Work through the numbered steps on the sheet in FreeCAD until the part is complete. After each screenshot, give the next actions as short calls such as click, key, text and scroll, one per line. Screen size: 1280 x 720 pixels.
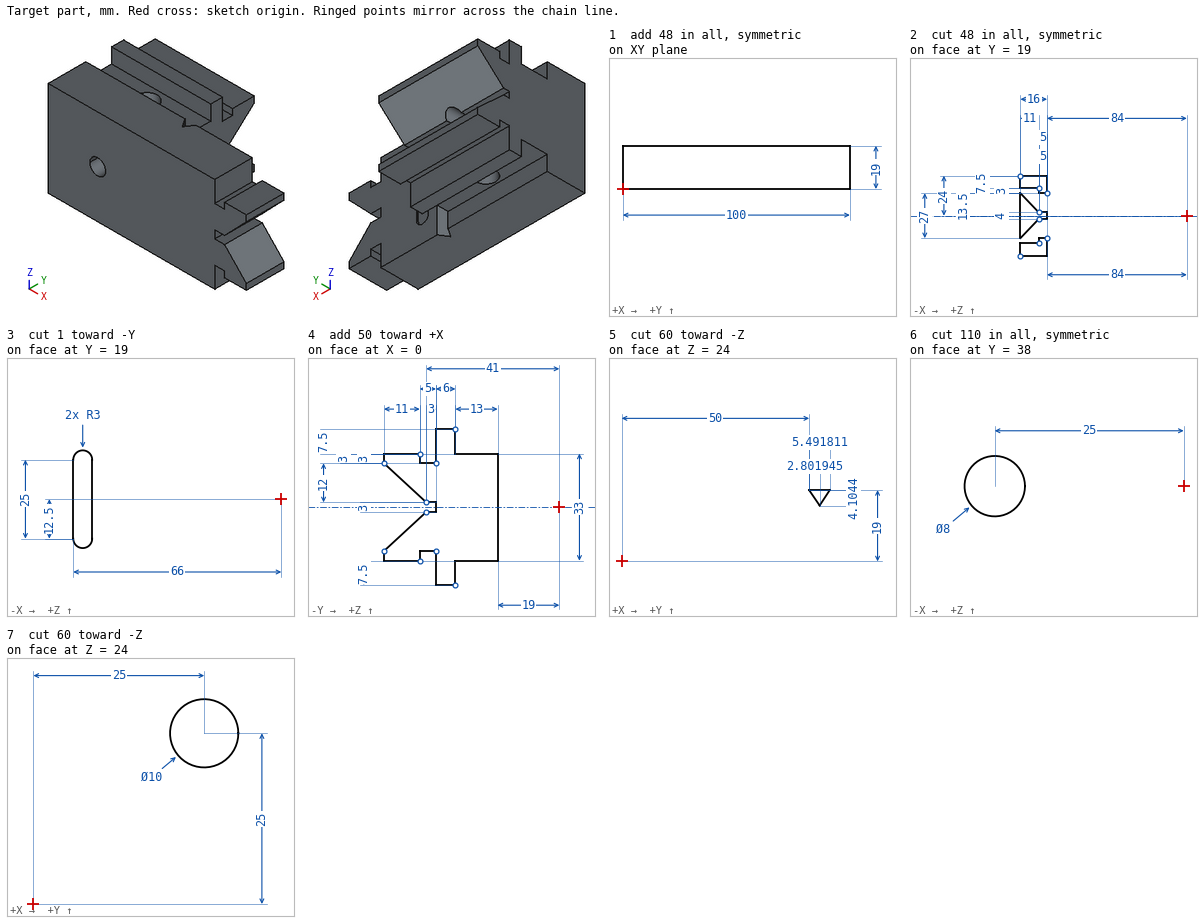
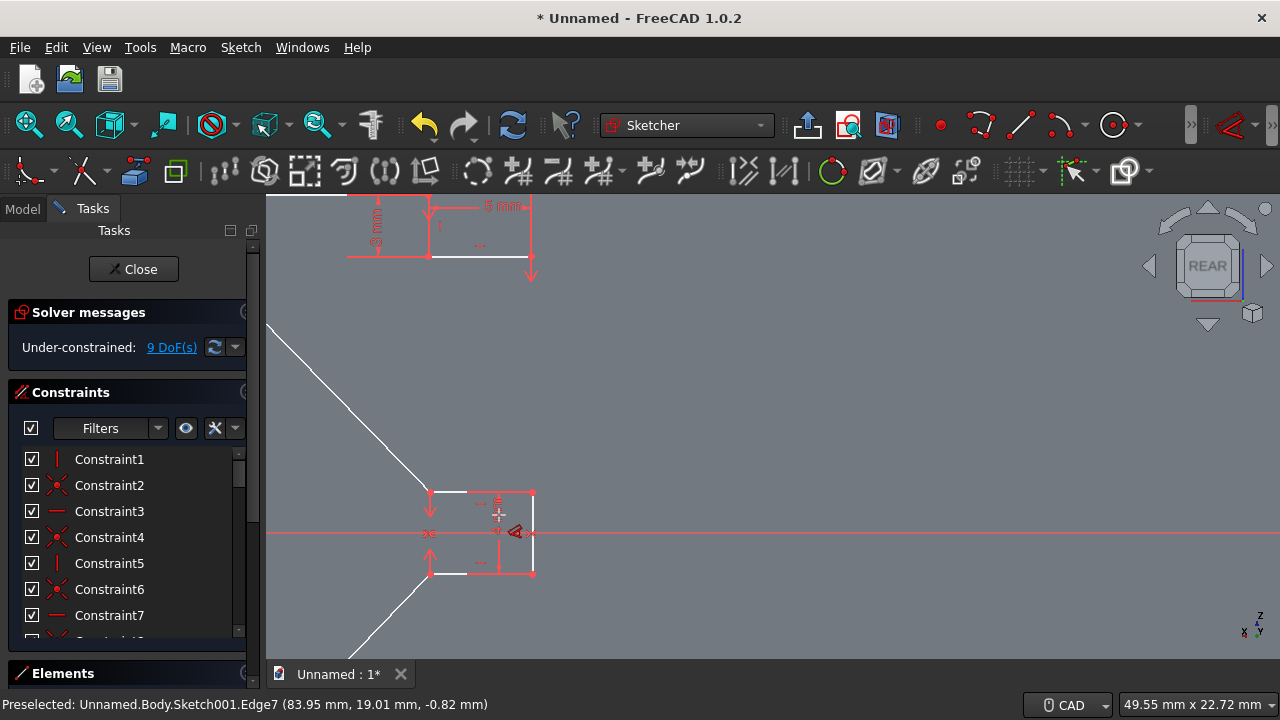
click(502, 492)
click(481, 458)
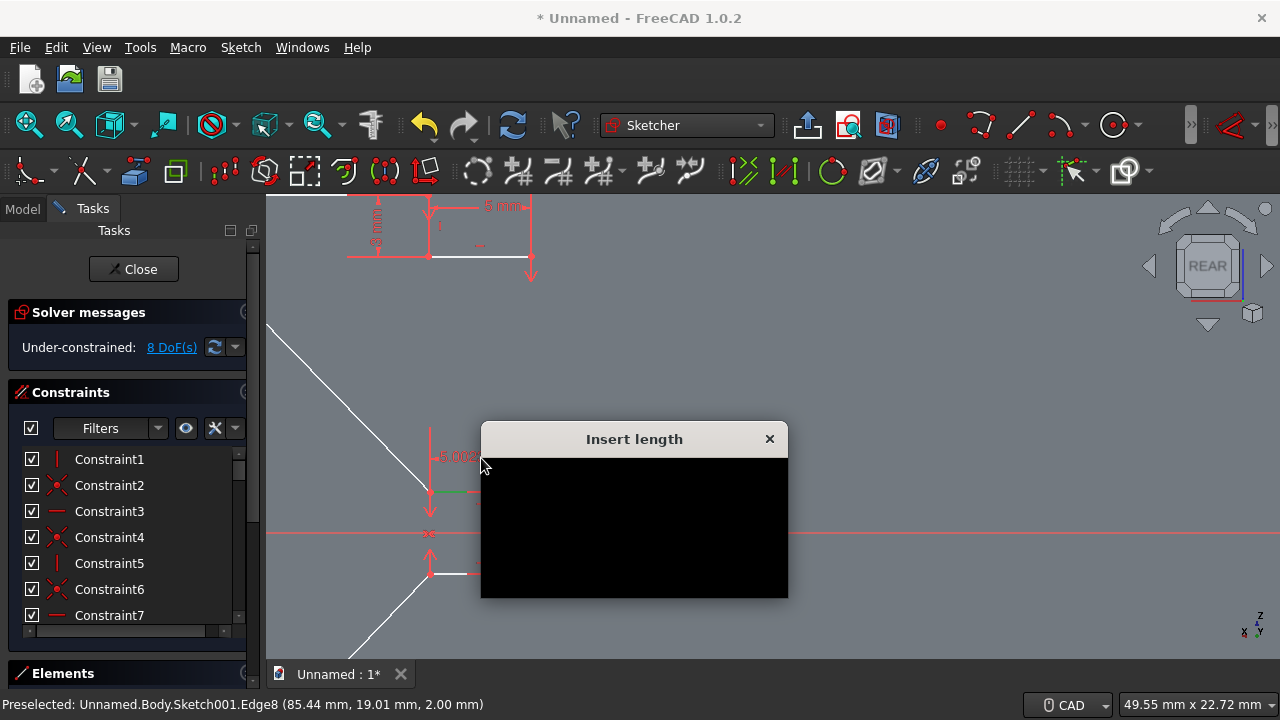
text(5)
key(Return)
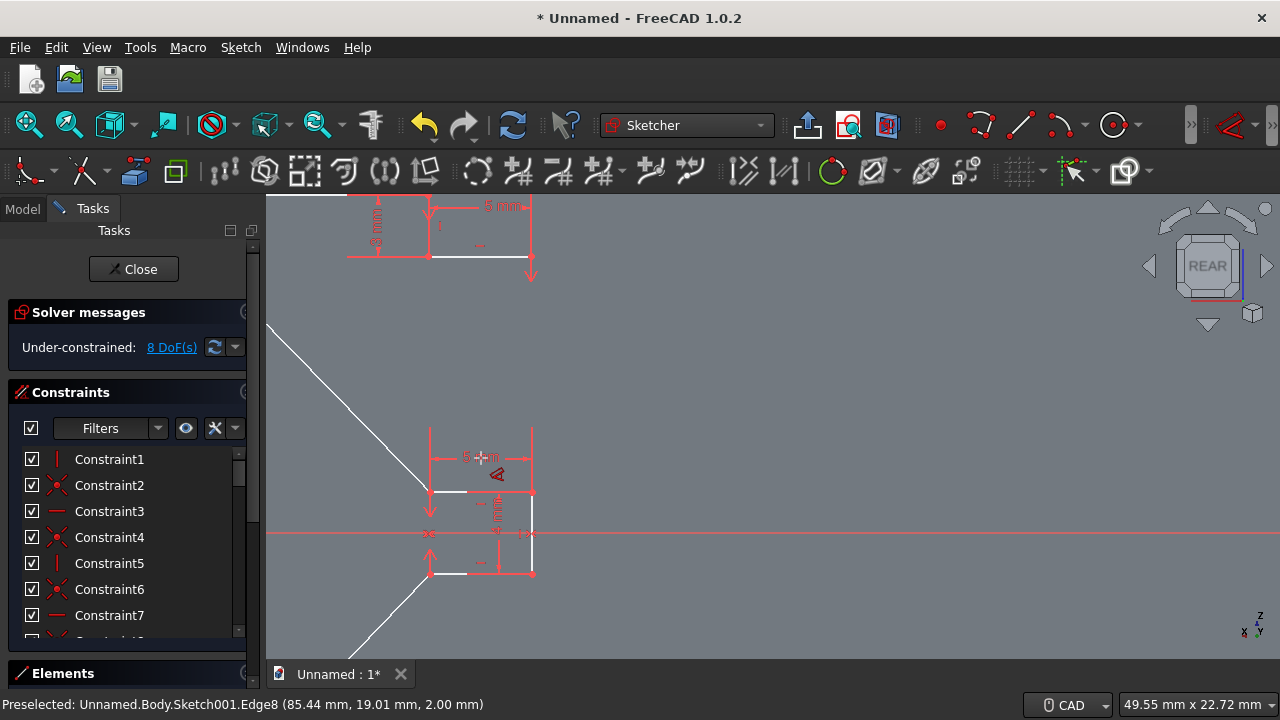
scroll(479, 381, down, 6)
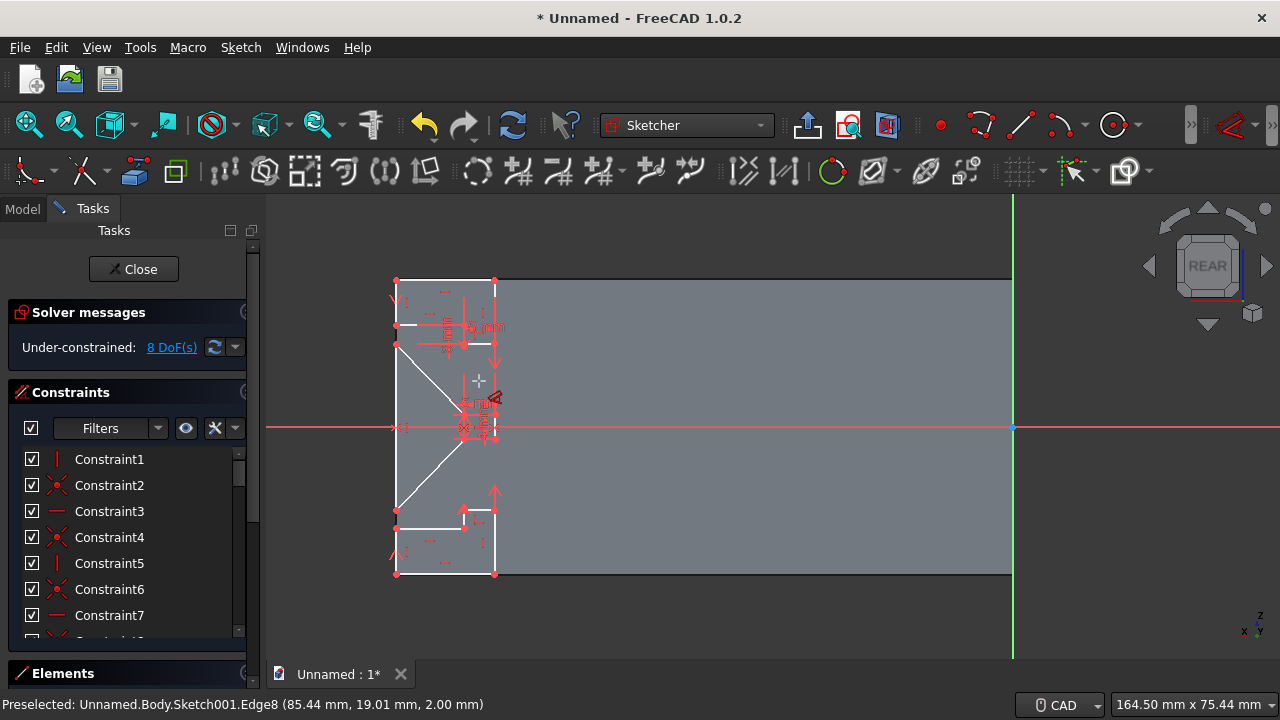
click(465, 280)
click(445, 246)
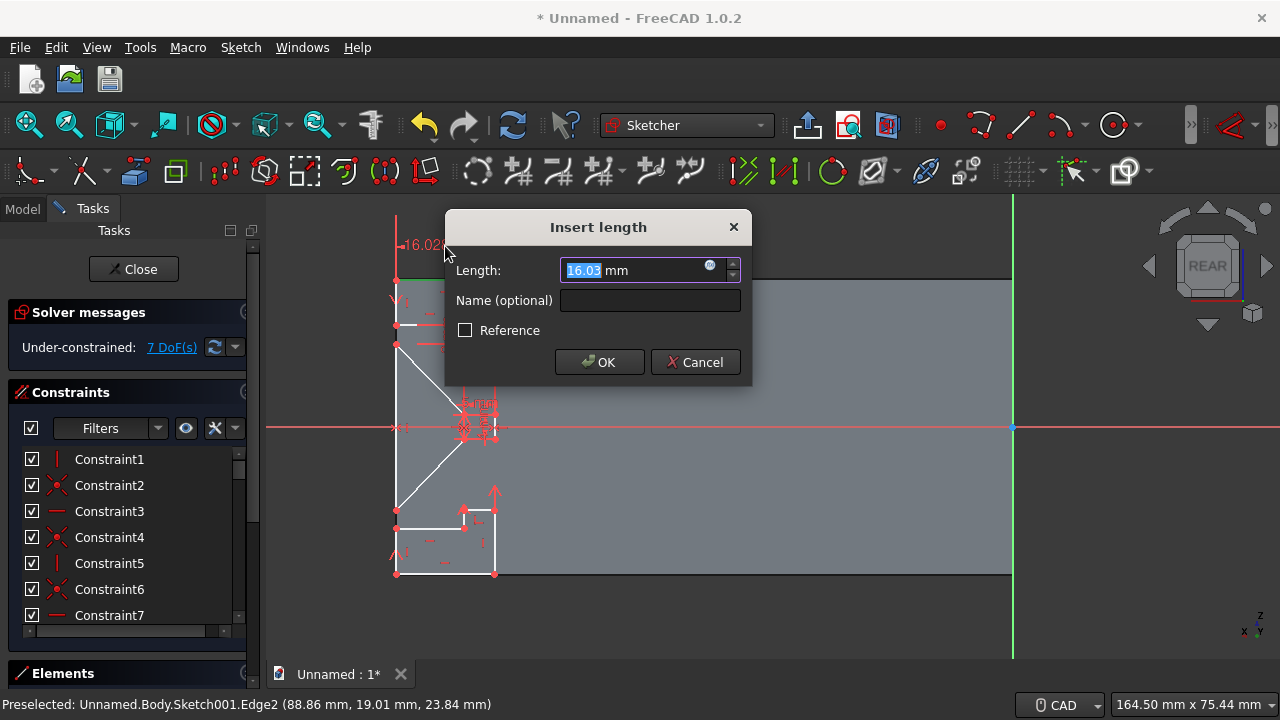
text(16)
key(Return)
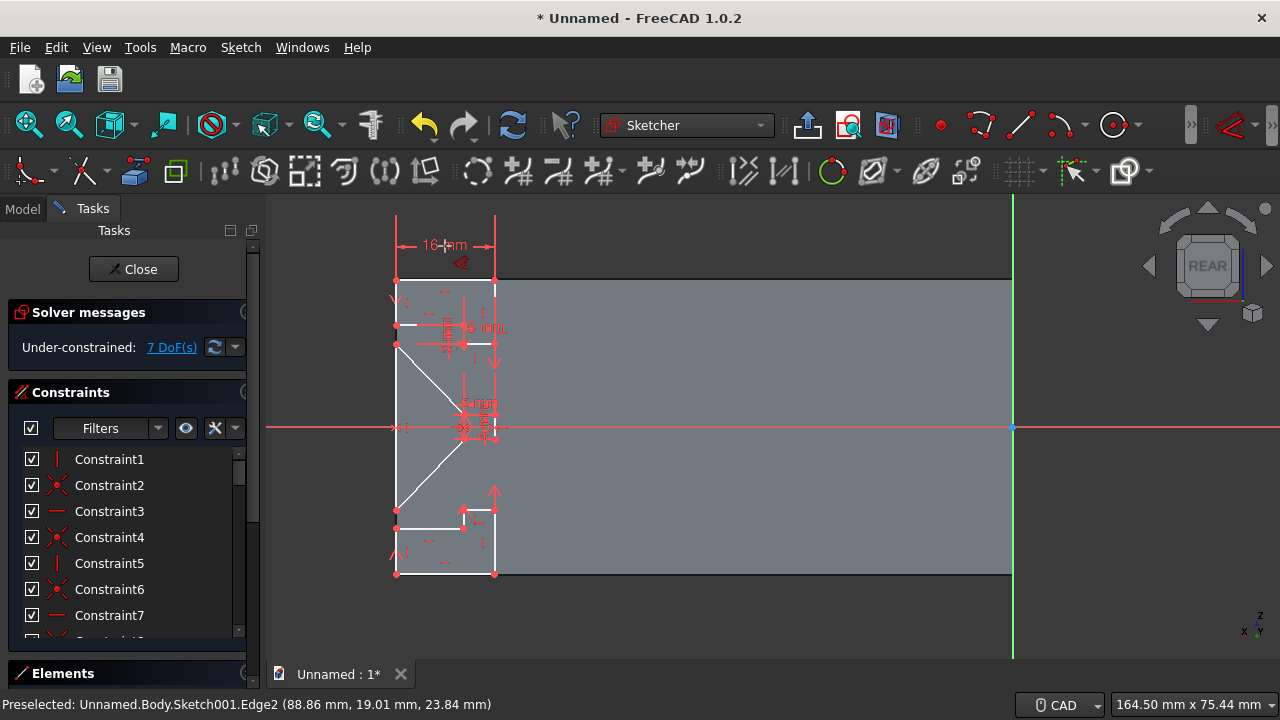
click(396, 394)
click(362, 390)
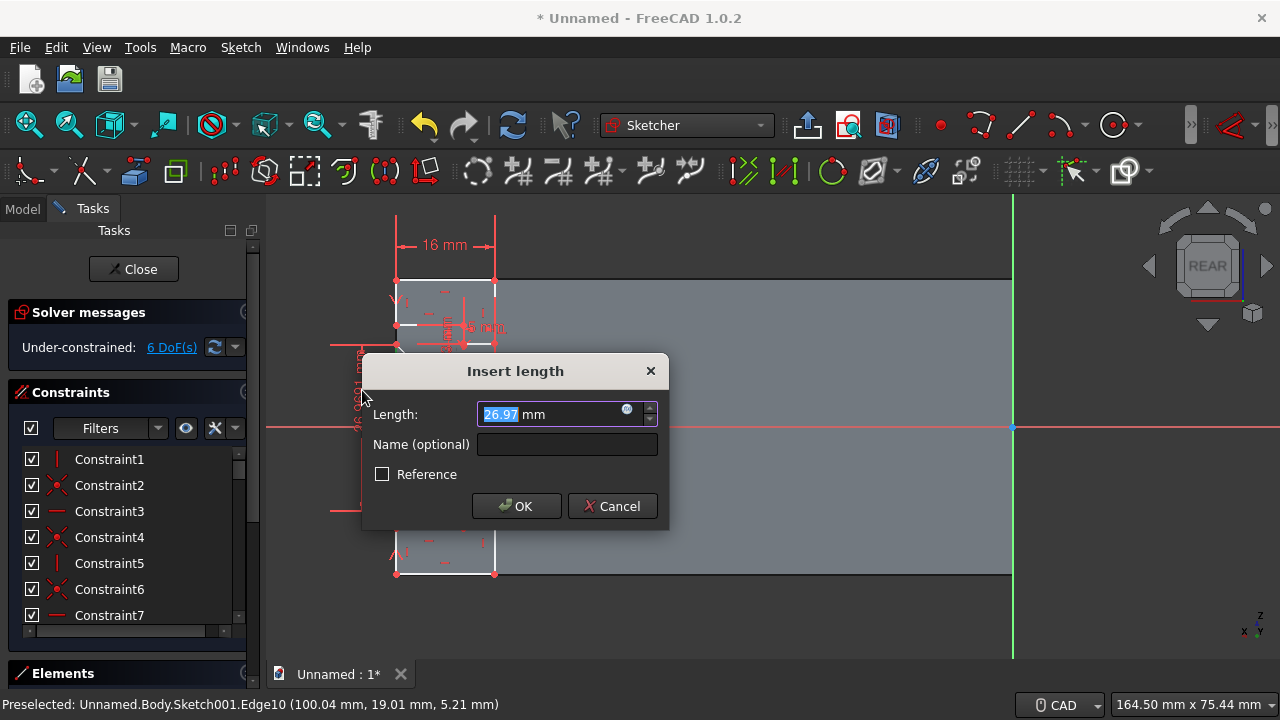
text(27)
key(Return)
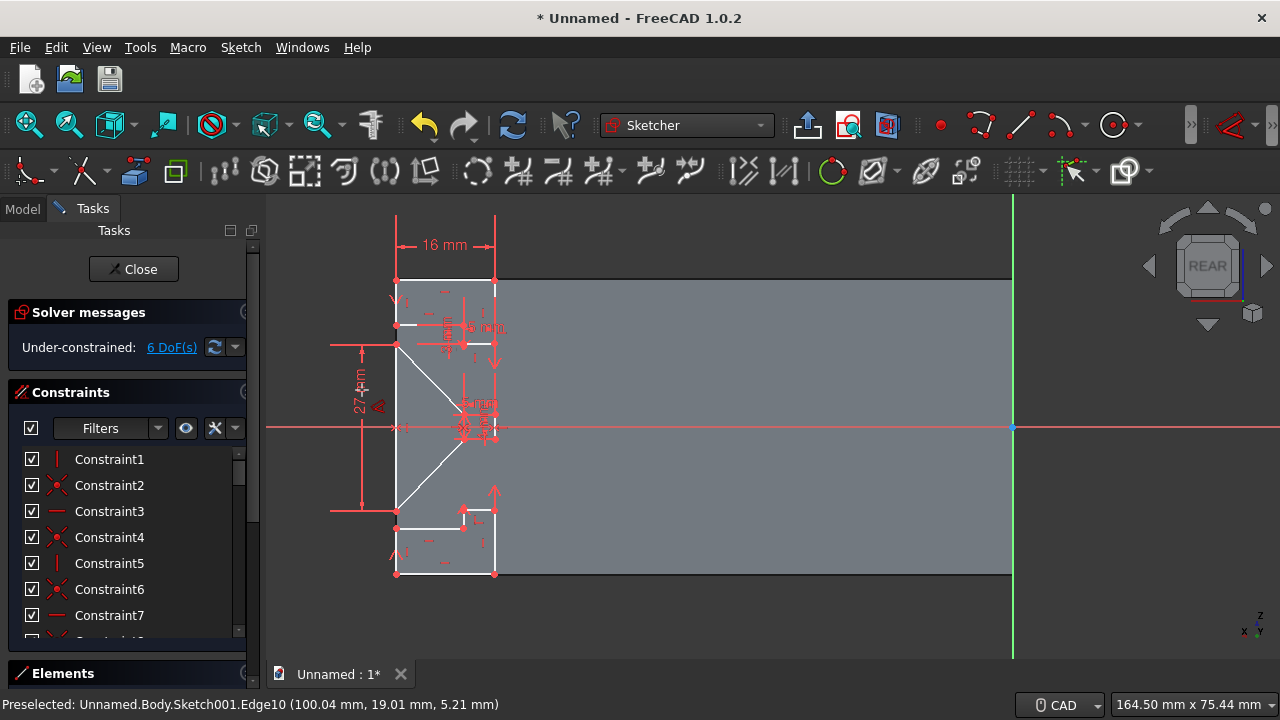
click(396, 294)
click(362, 303)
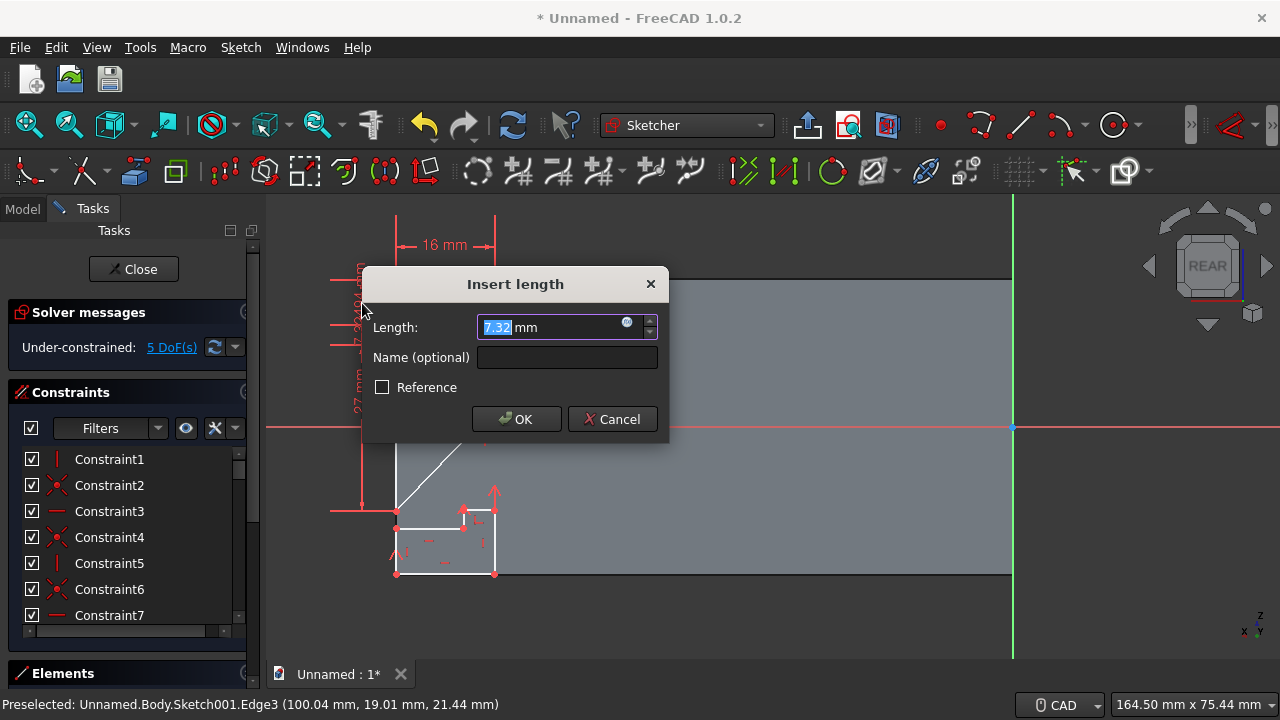
text(7.5)
key(Return)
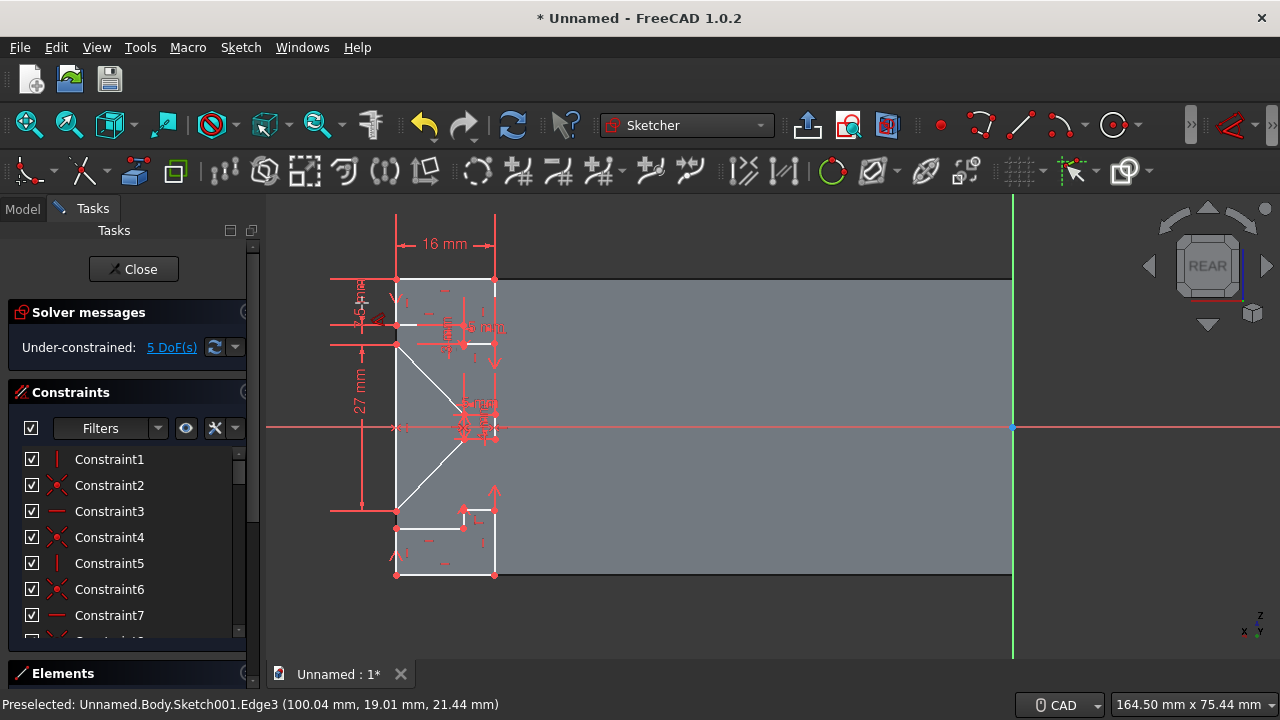
click(495, 344)
click(754, 310)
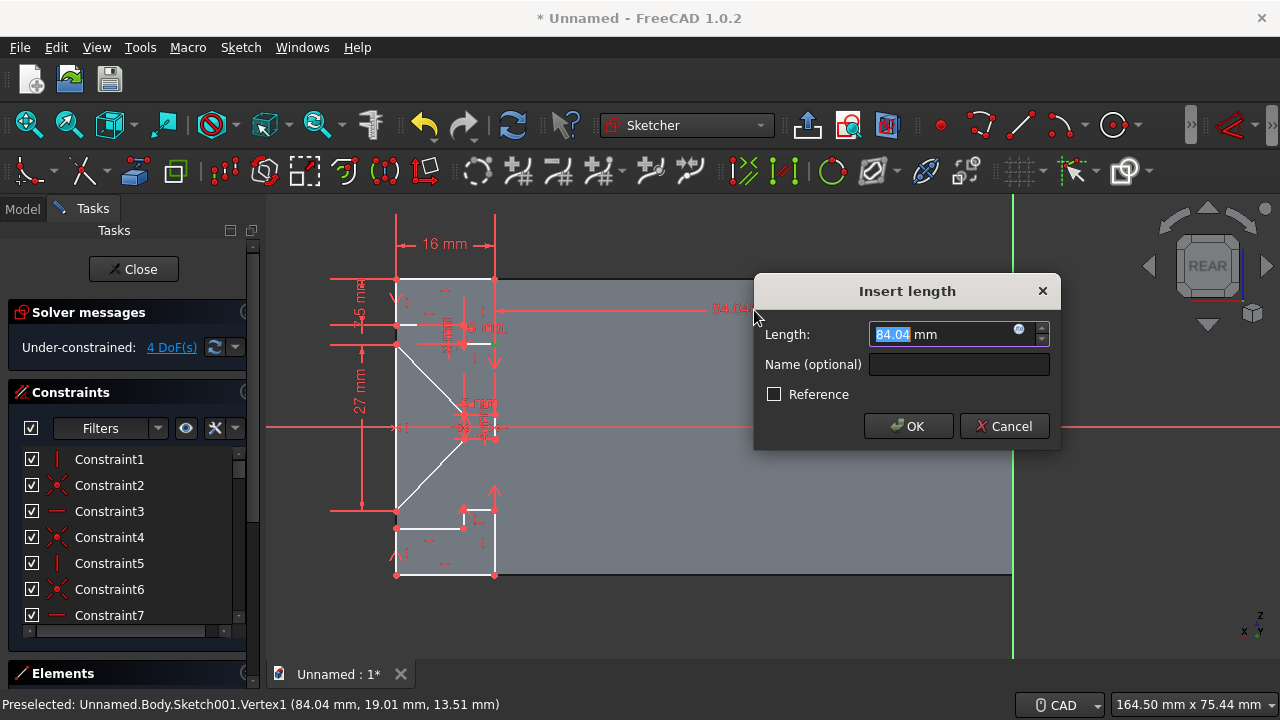
text(84)
key(Return)